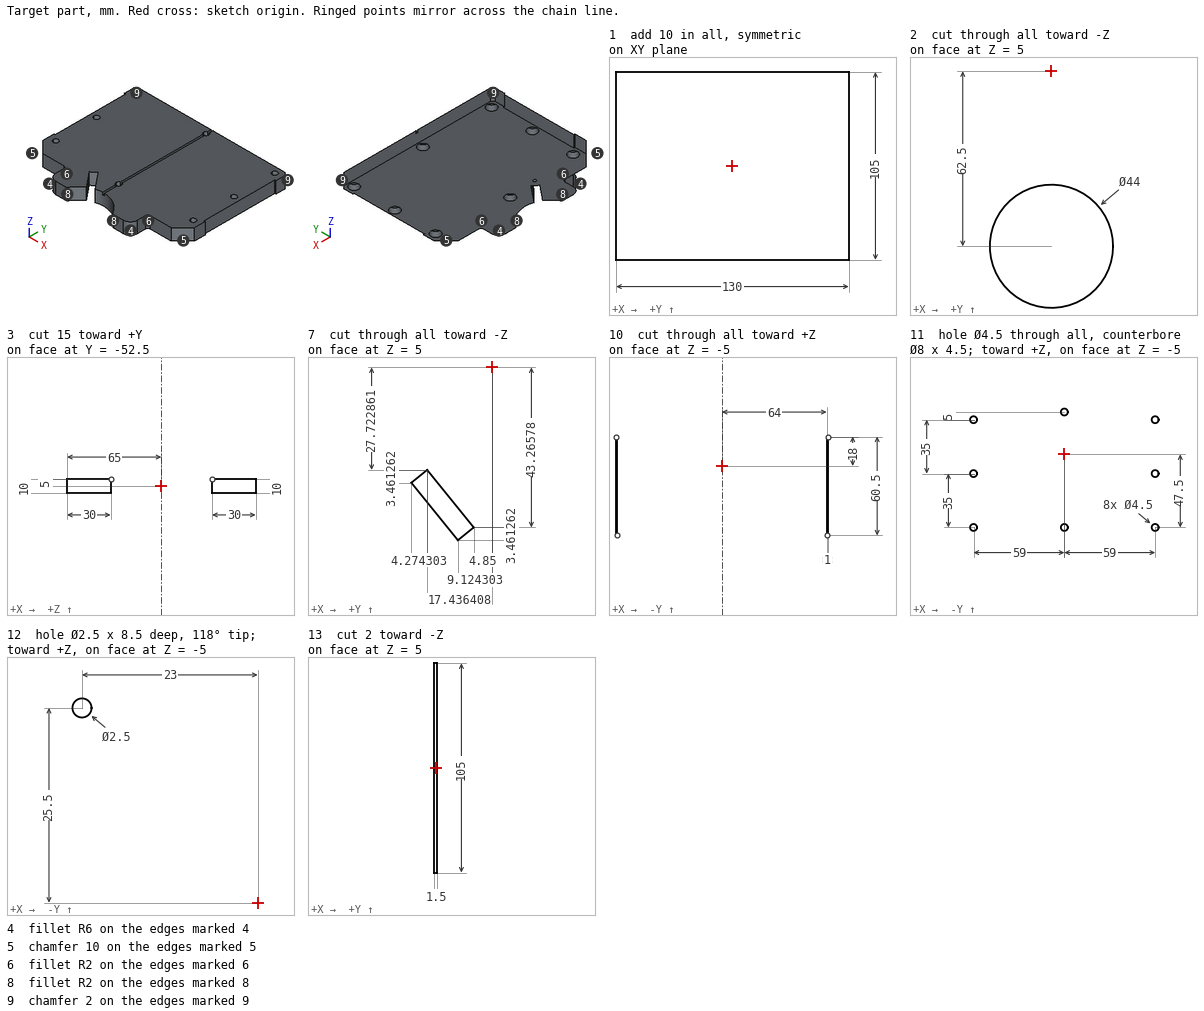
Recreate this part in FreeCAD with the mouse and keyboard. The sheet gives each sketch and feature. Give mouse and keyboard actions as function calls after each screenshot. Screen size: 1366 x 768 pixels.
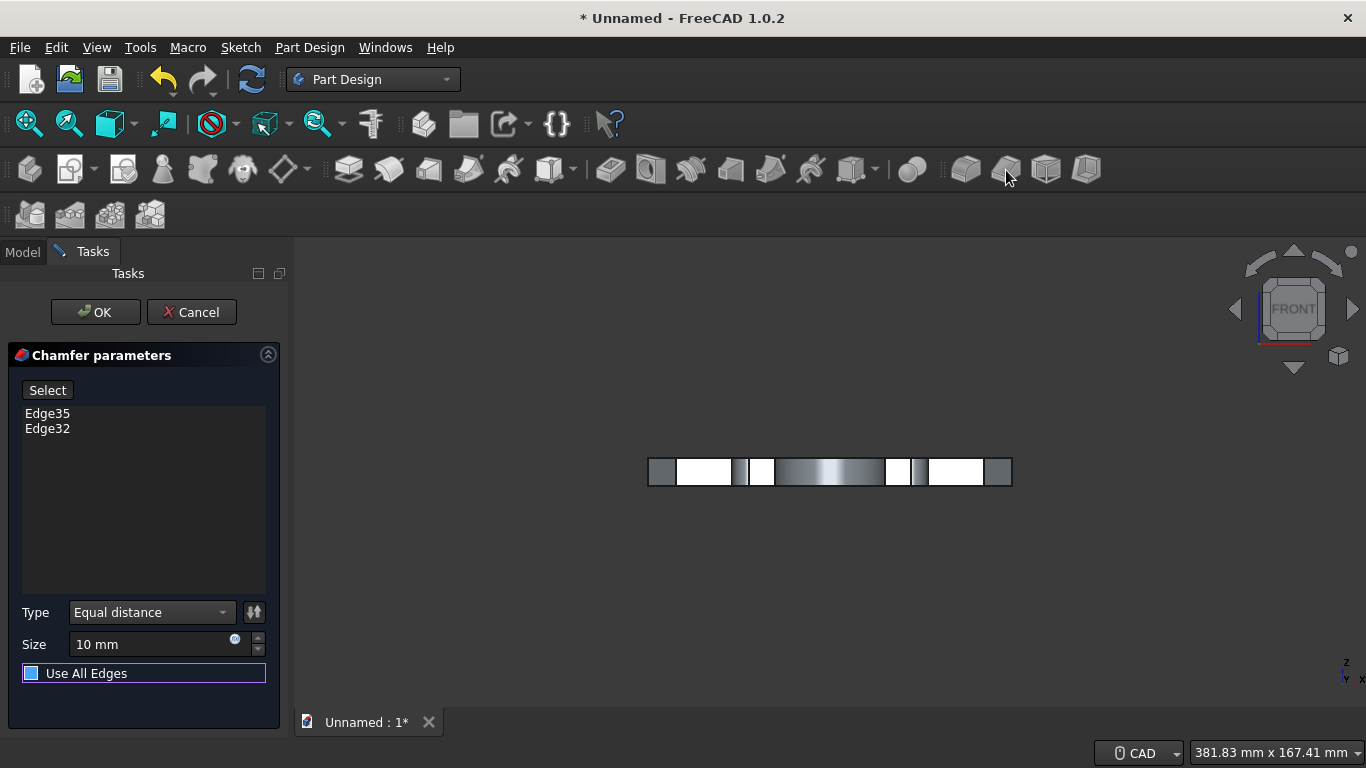
click(96, 312)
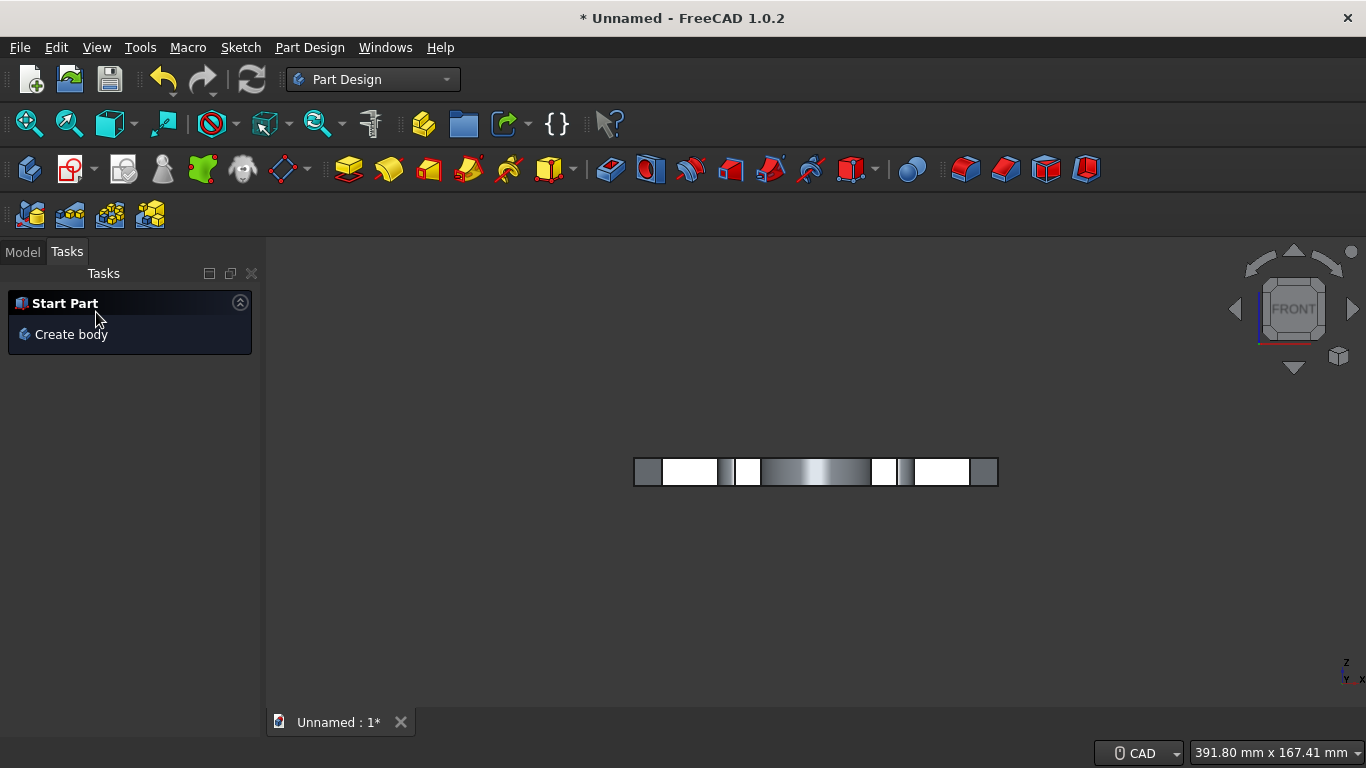
click(30, 124)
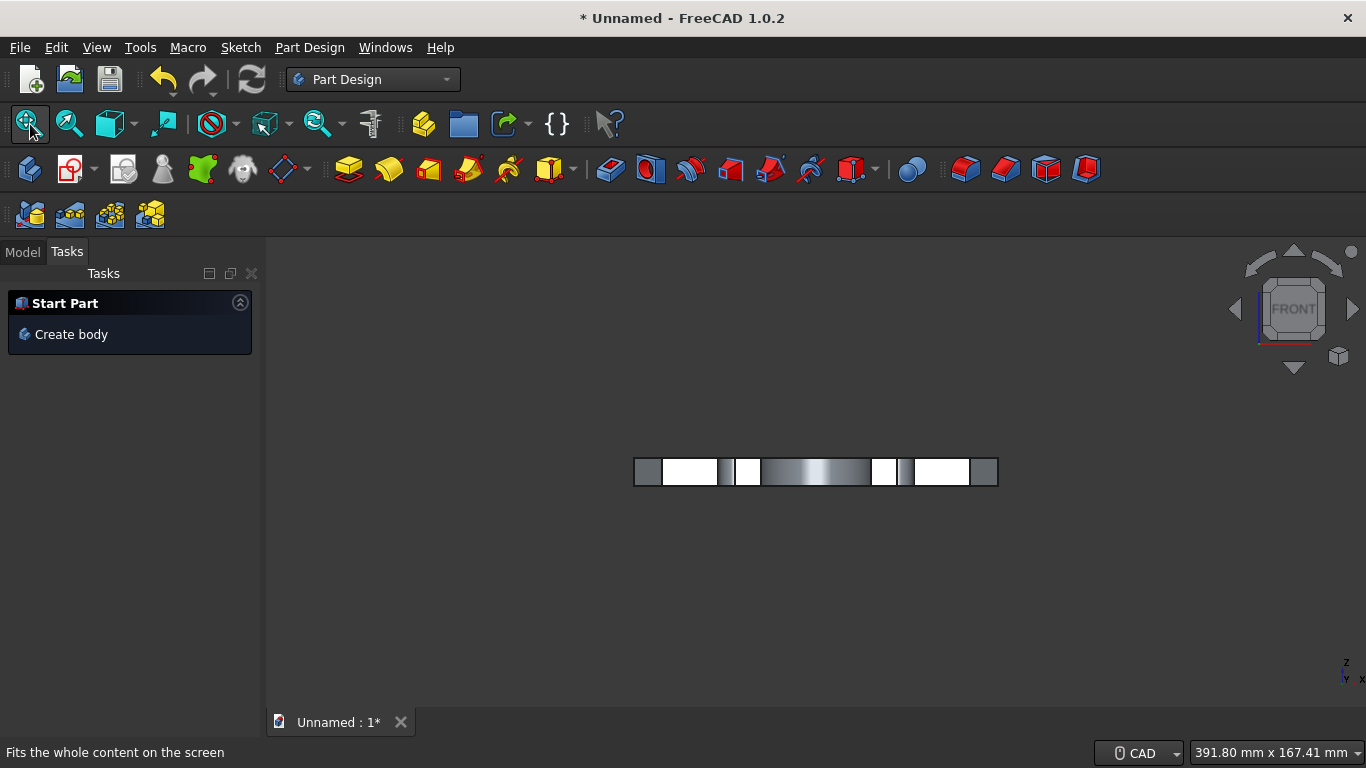
key(0)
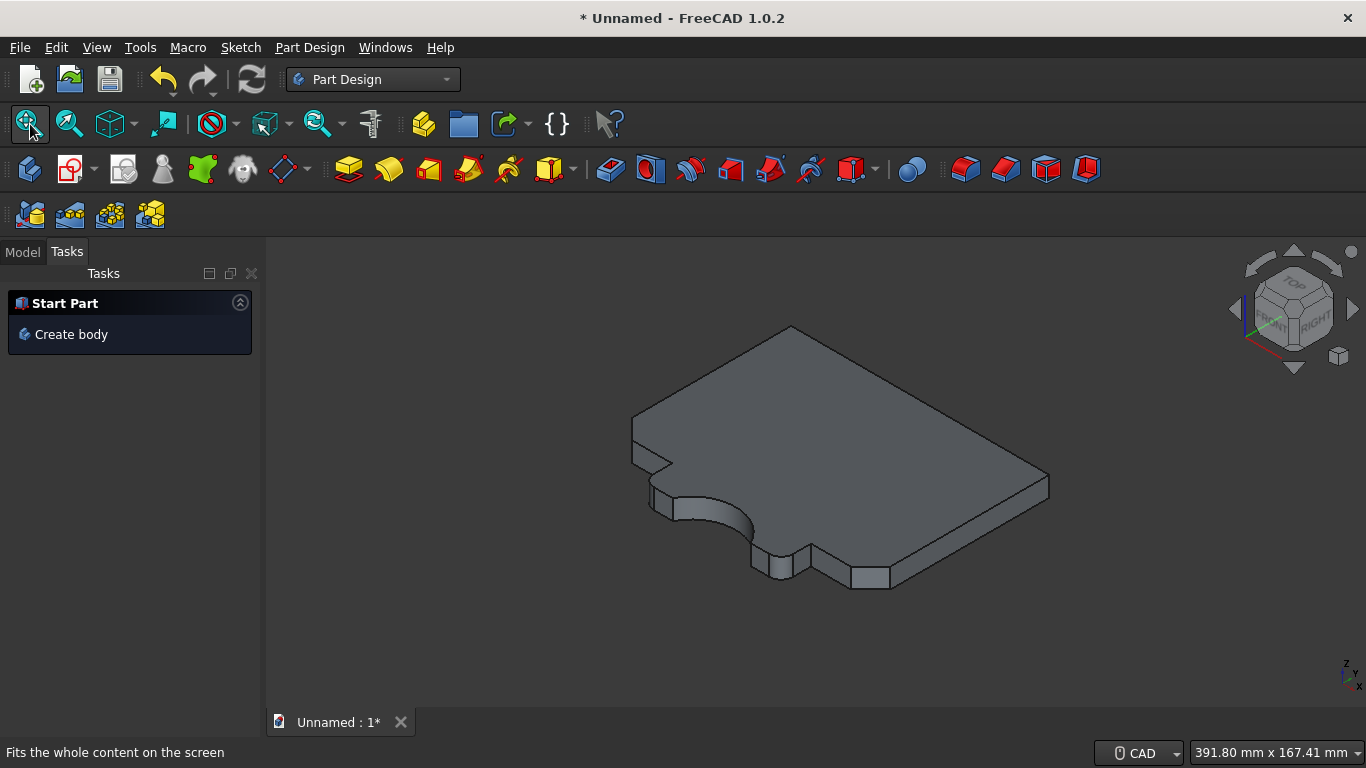
key(2)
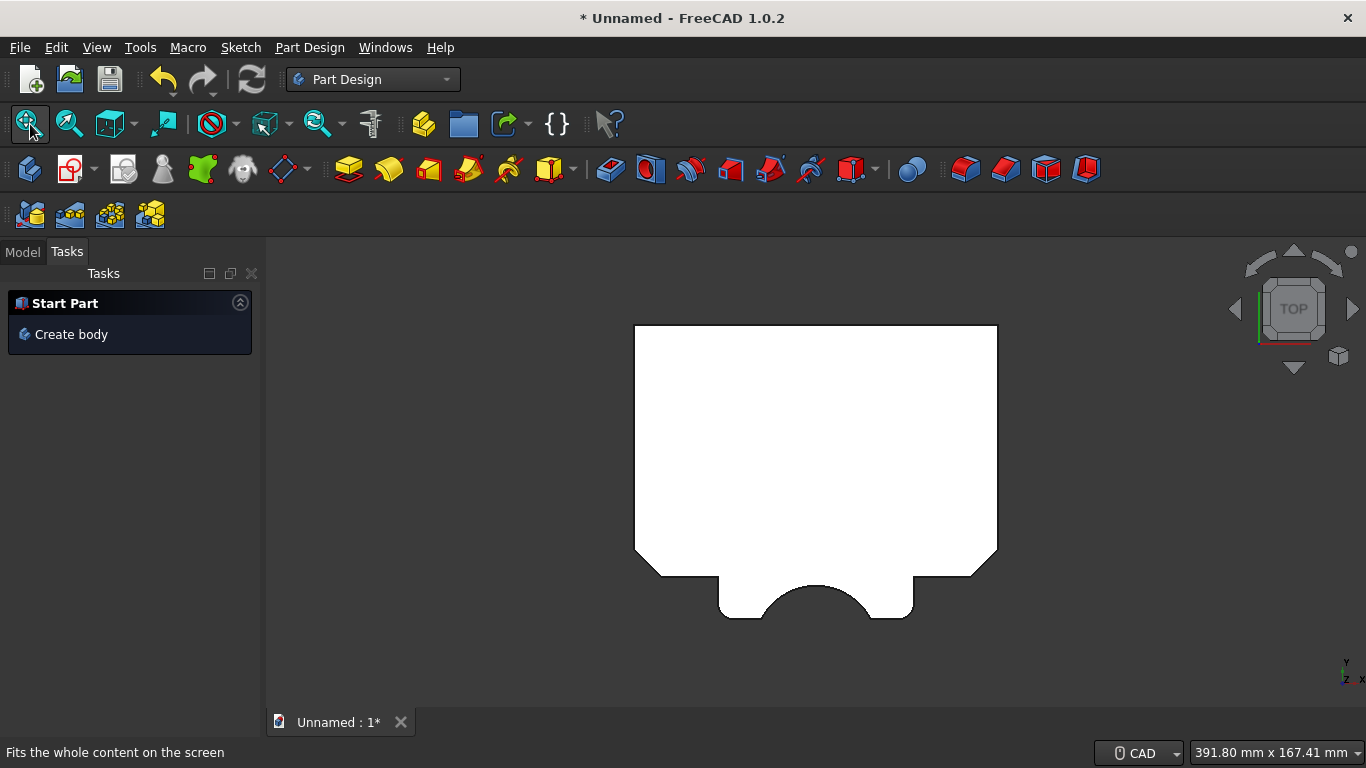
key(1)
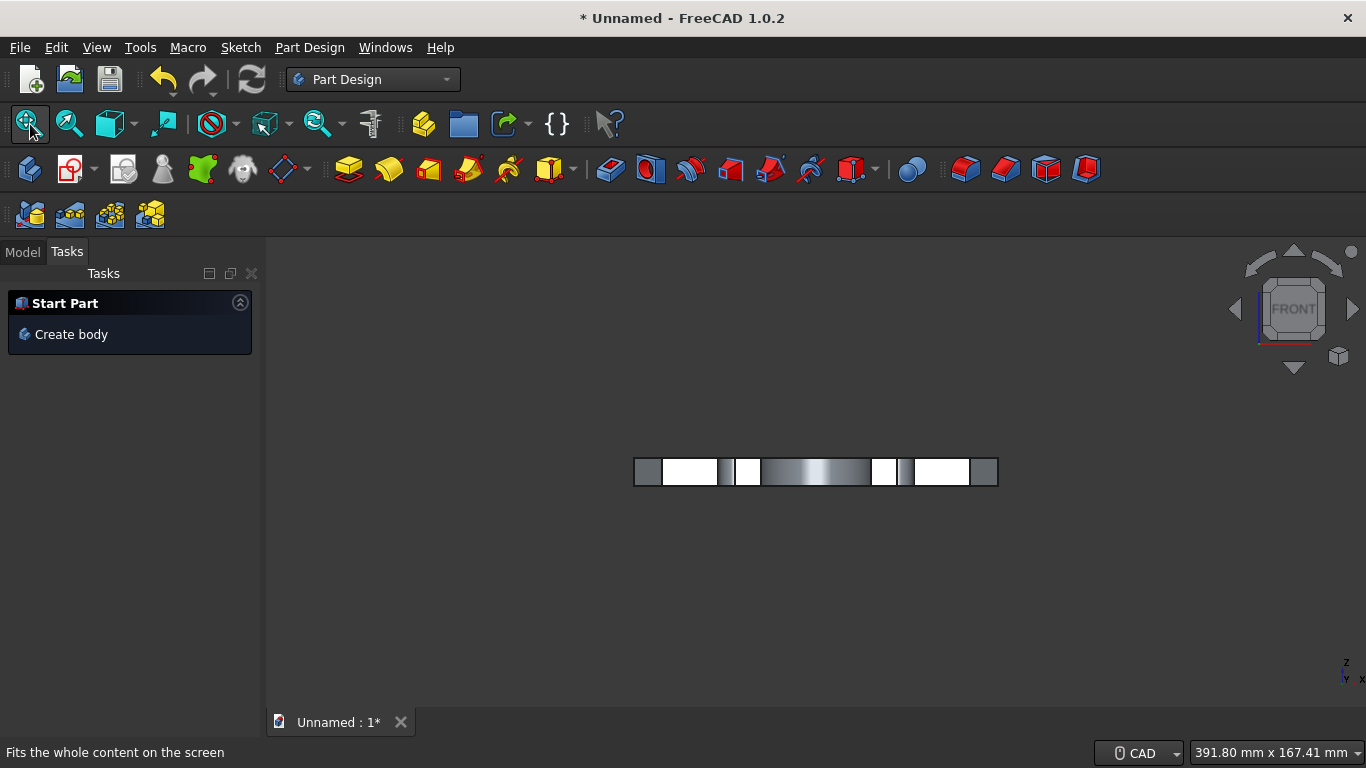
click(30, 124)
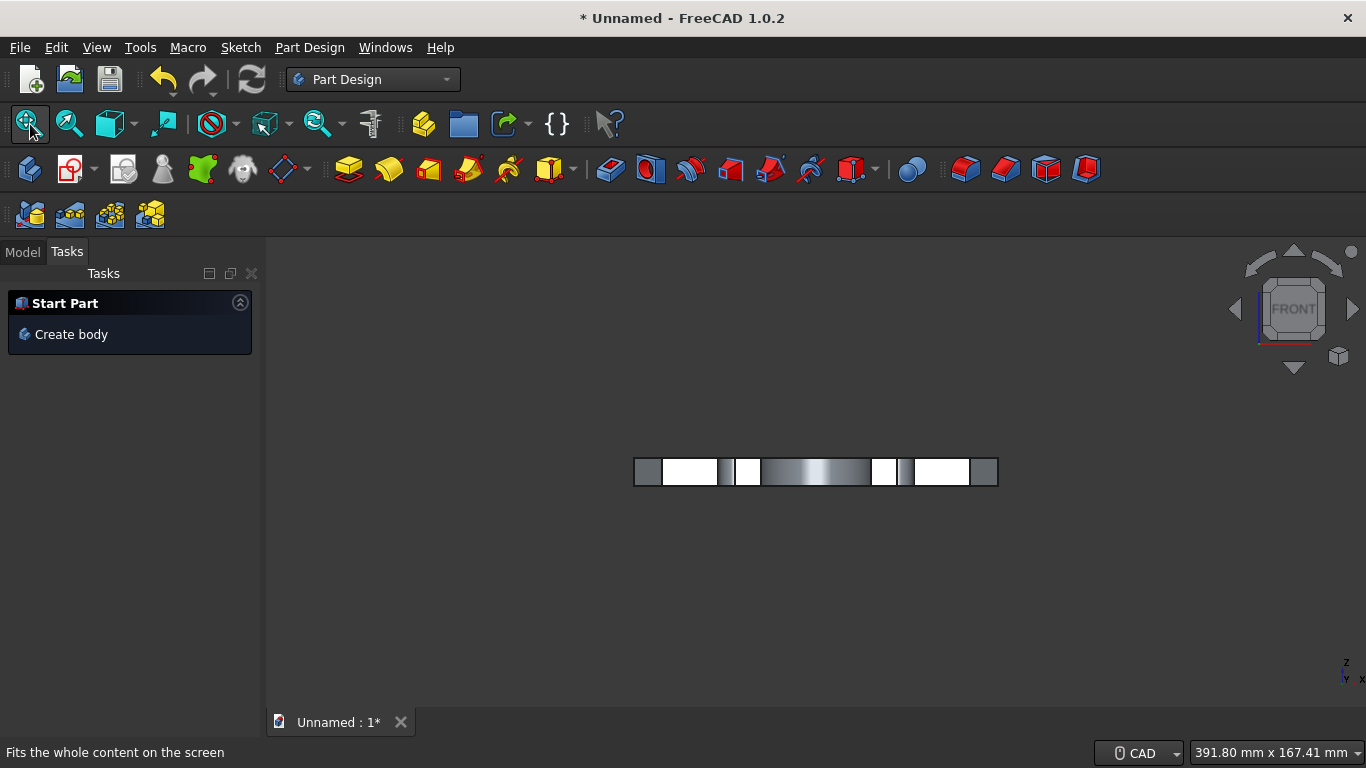
key(3)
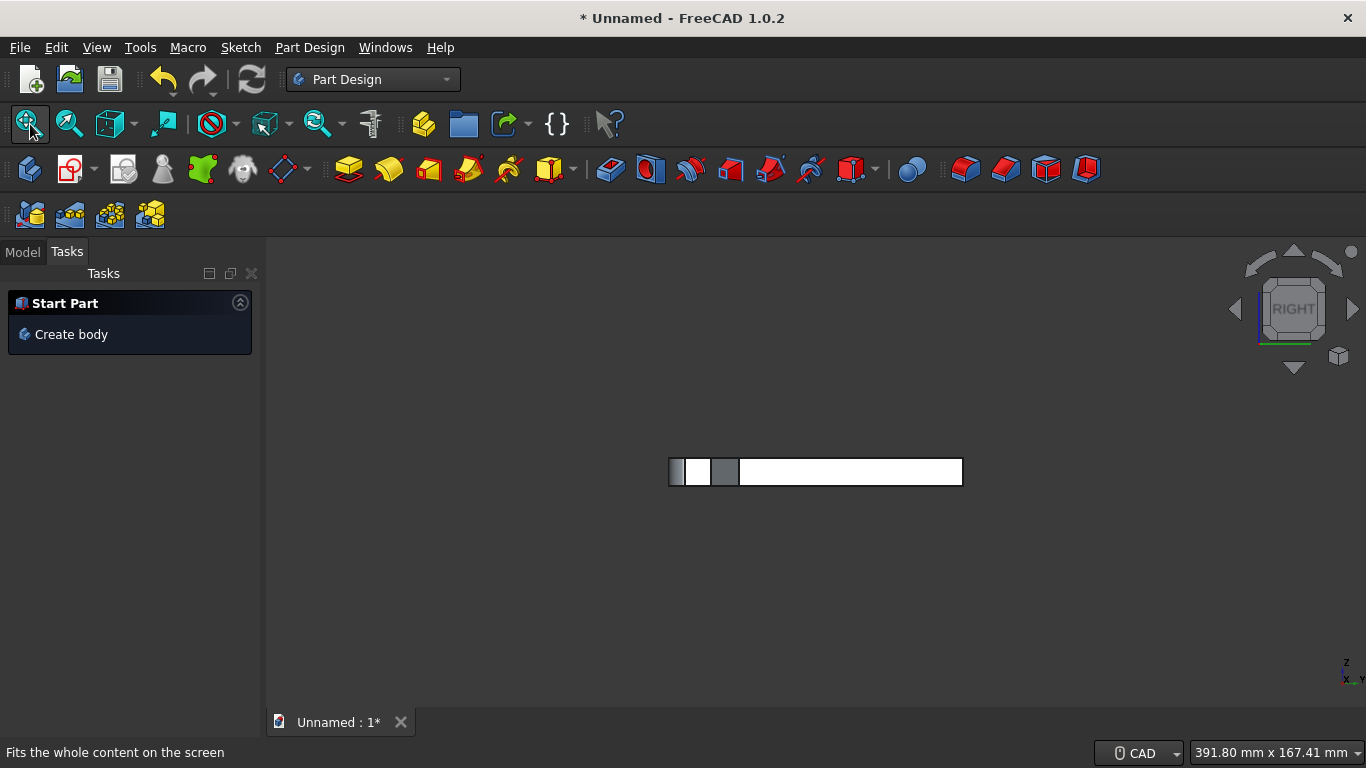
click(30, 124)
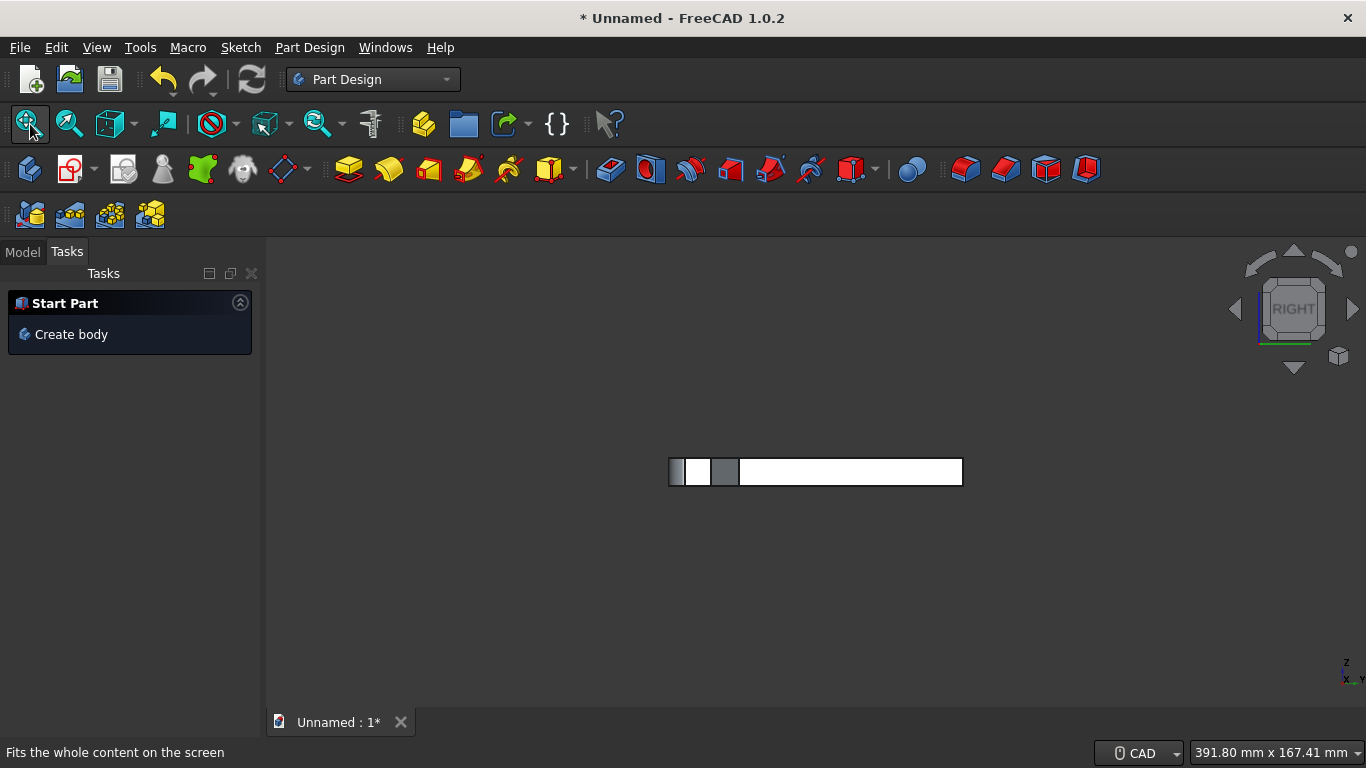
key(5)